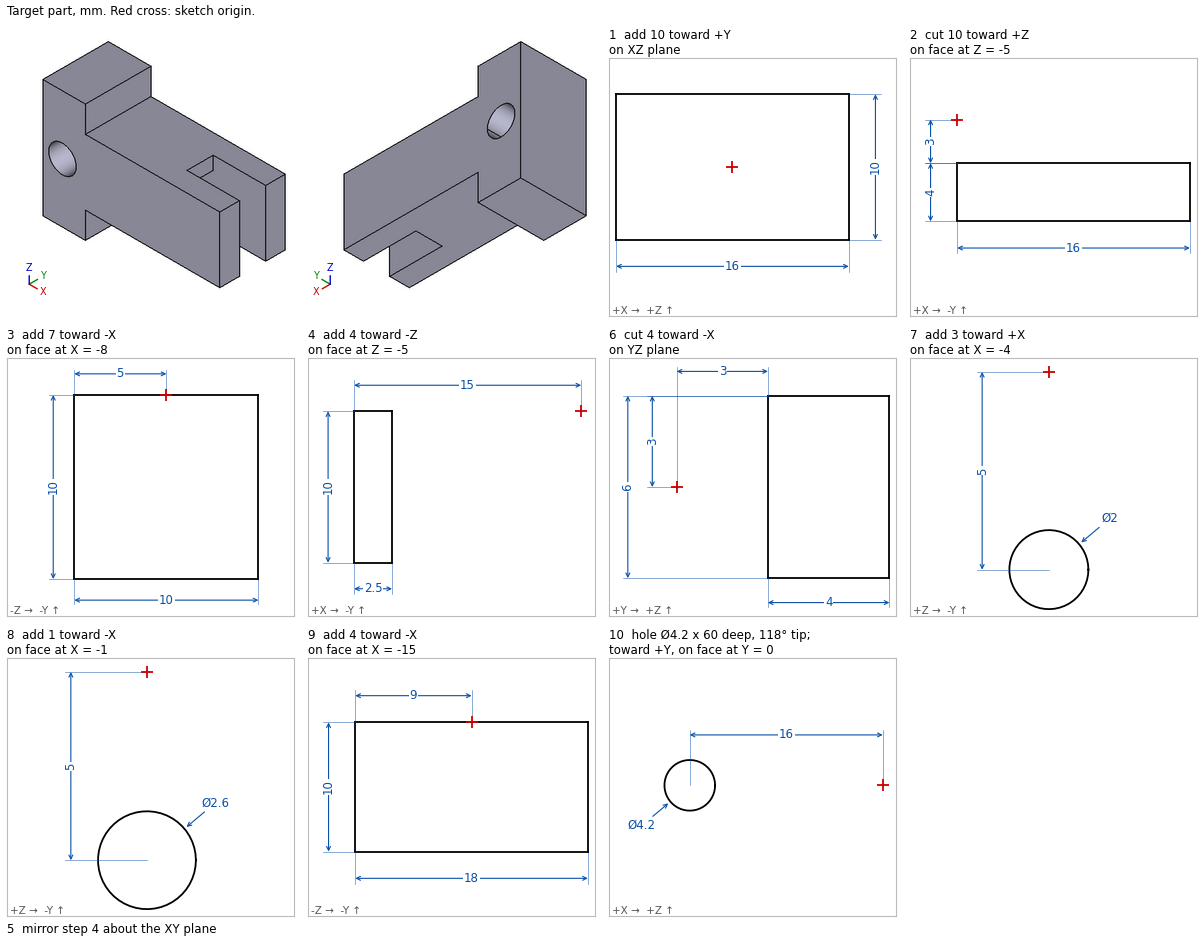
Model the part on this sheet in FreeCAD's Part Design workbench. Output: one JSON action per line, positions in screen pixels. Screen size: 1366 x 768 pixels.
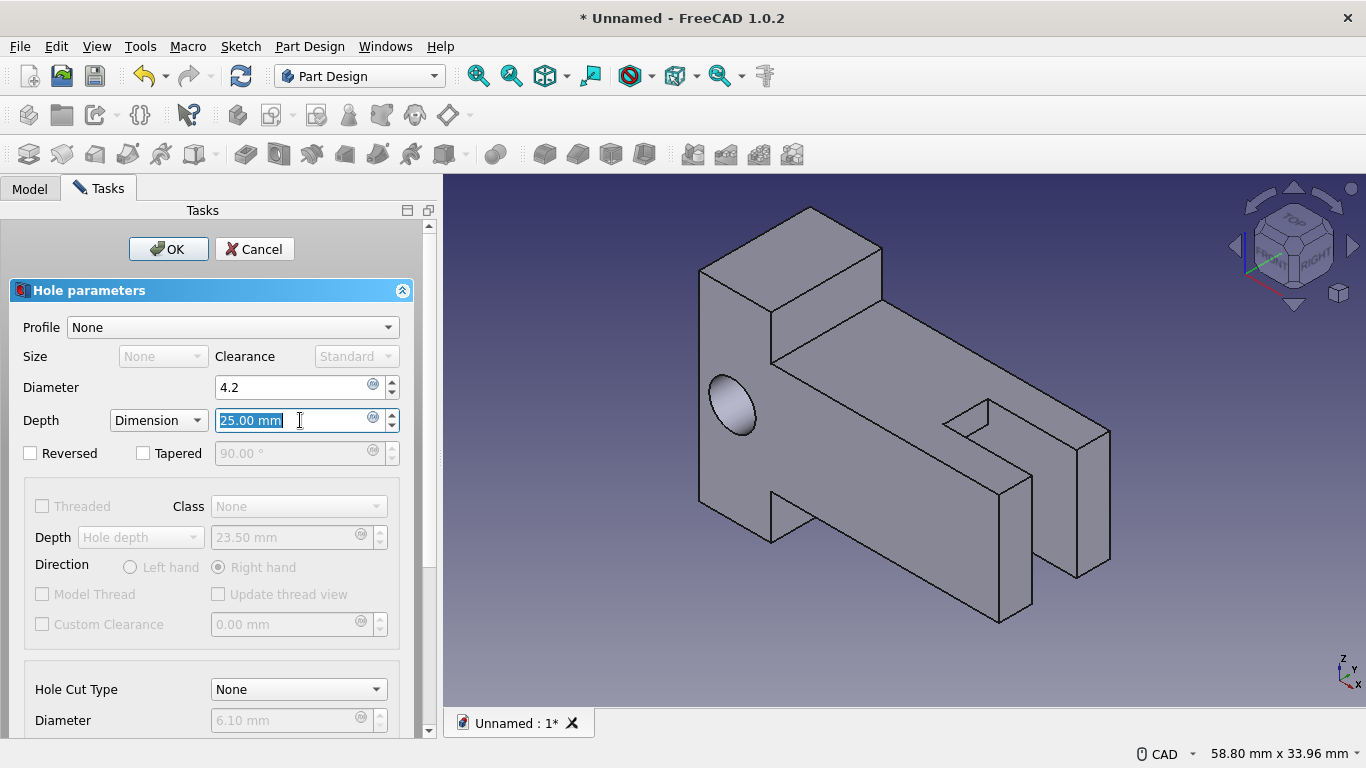
{"action": "type", "text": "60"}
{"action": "key", "text": "Tab"}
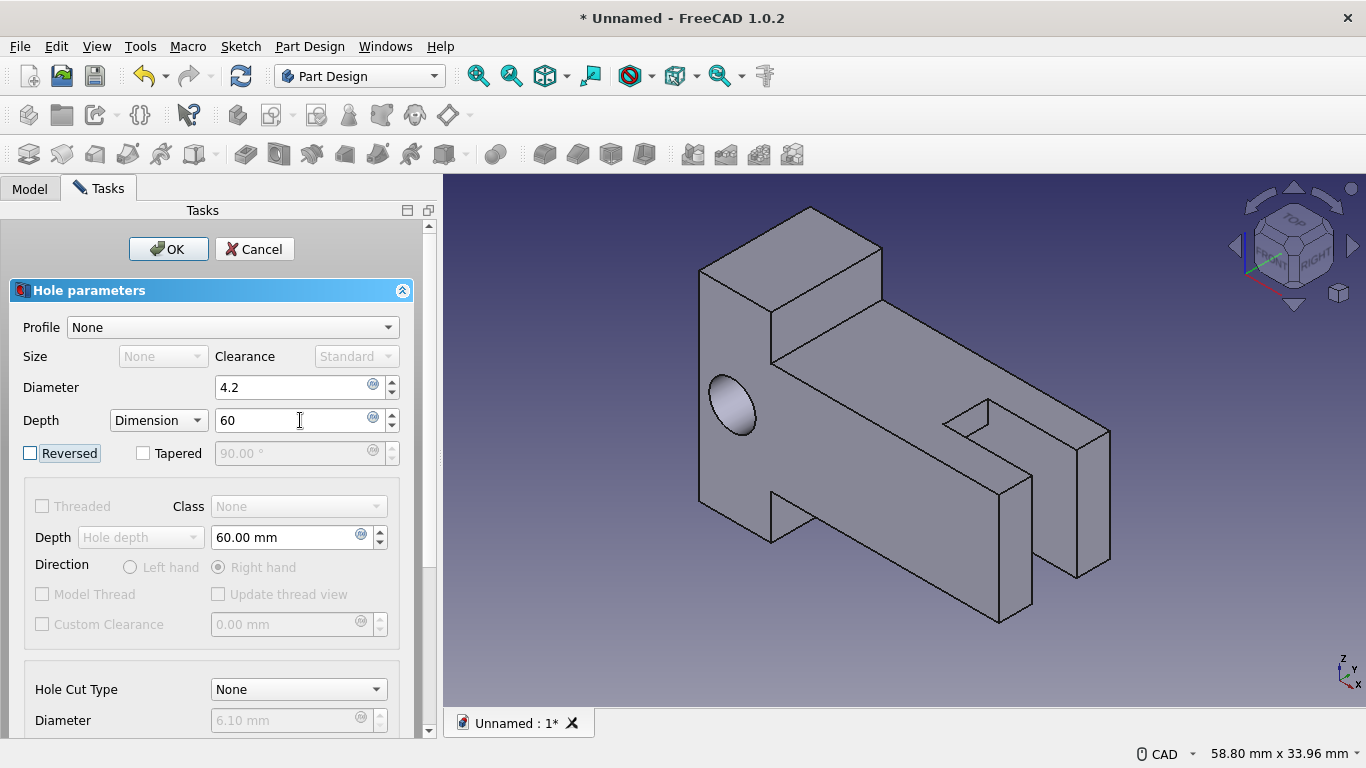
{"action": "left_click", "coordinate": [169, 249]}